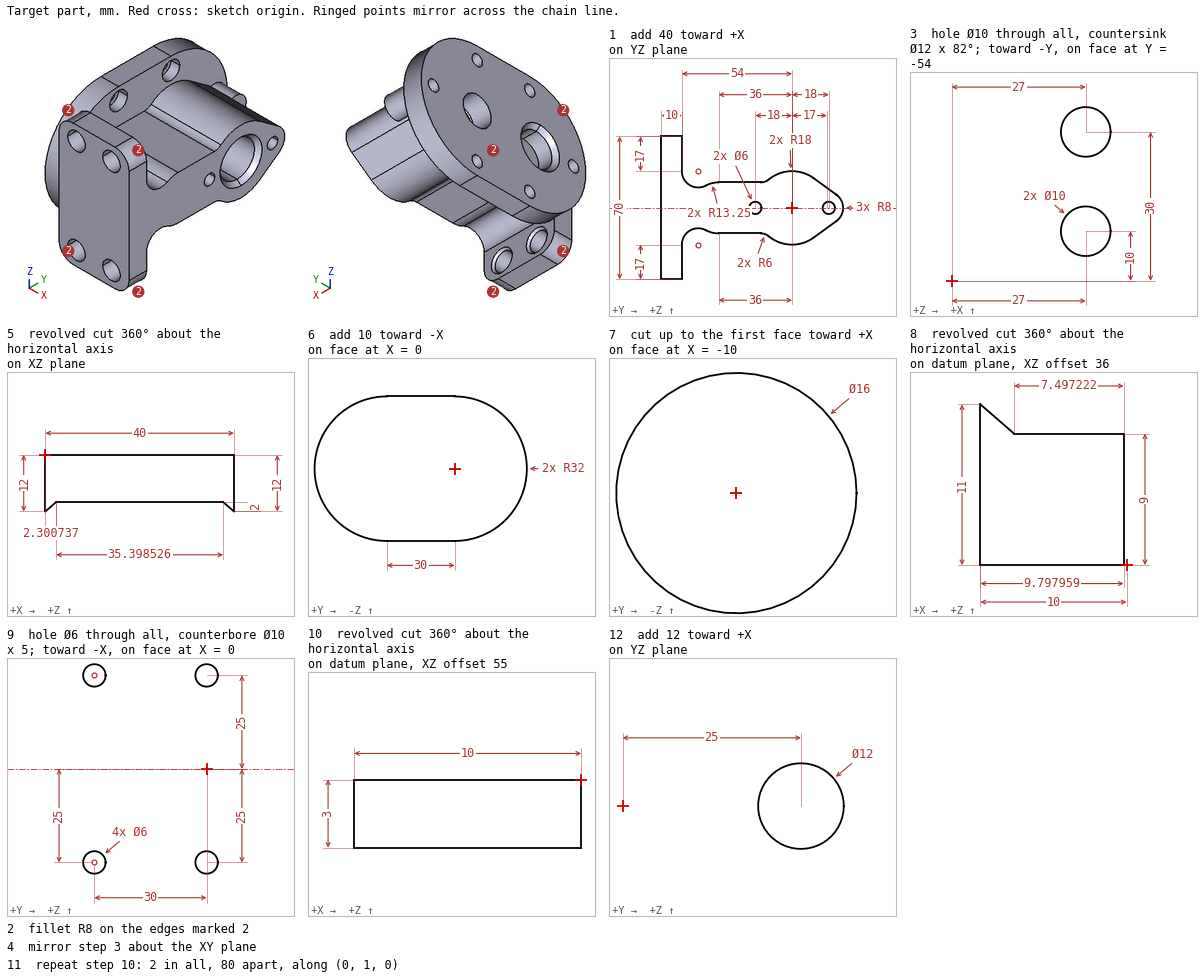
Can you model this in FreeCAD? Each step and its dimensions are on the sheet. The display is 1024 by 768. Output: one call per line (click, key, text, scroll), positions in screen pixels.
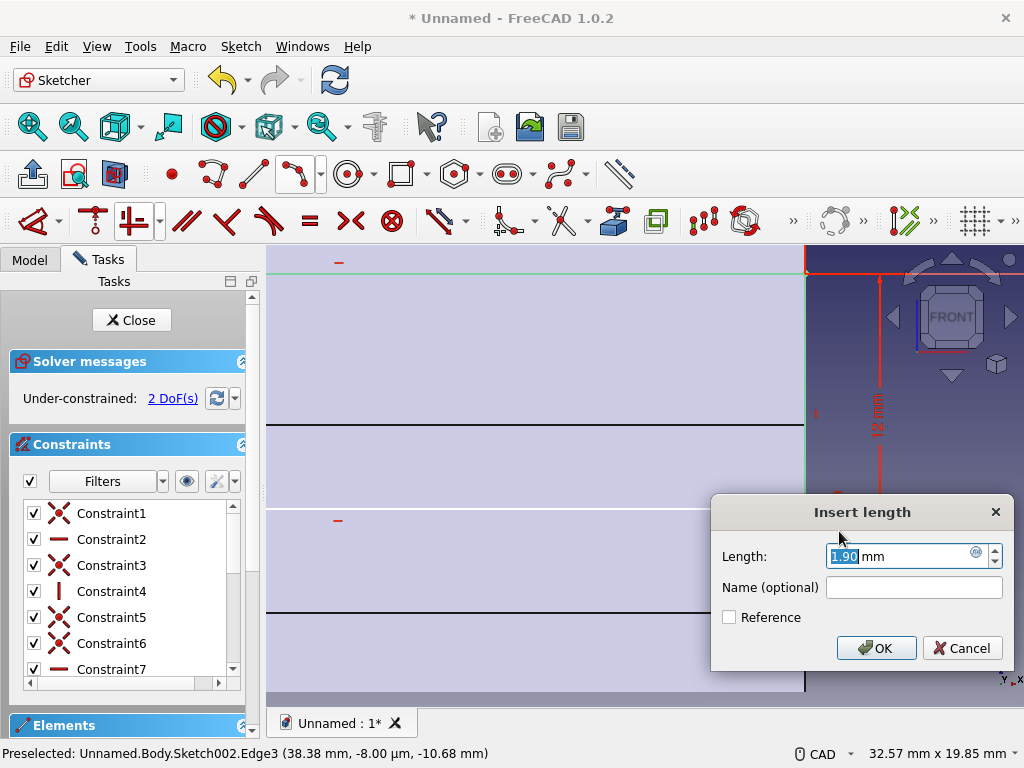
text(2)
key(Return)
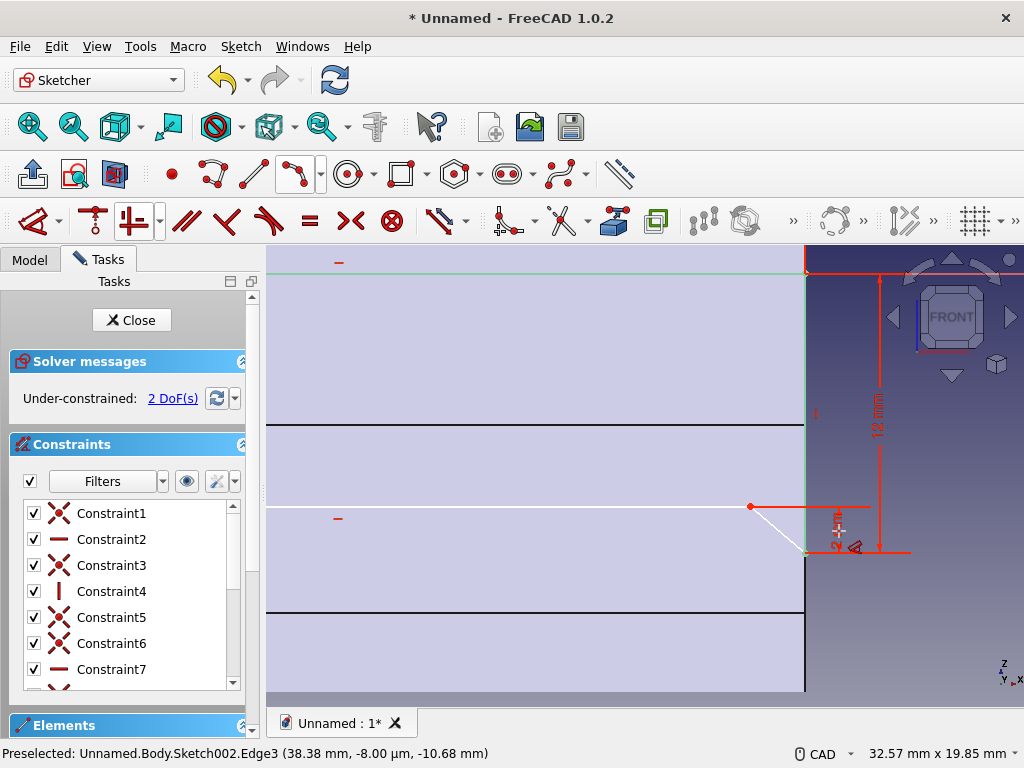
click(504, 507)
click(522, 541)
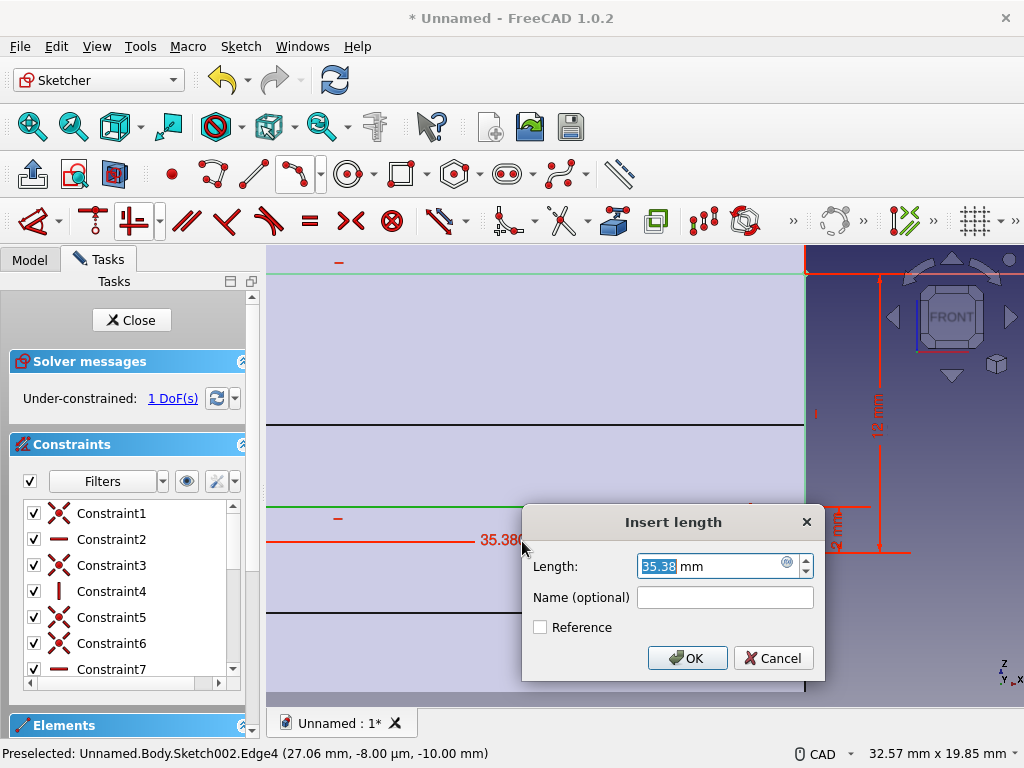
text(35.398526)
key(Return)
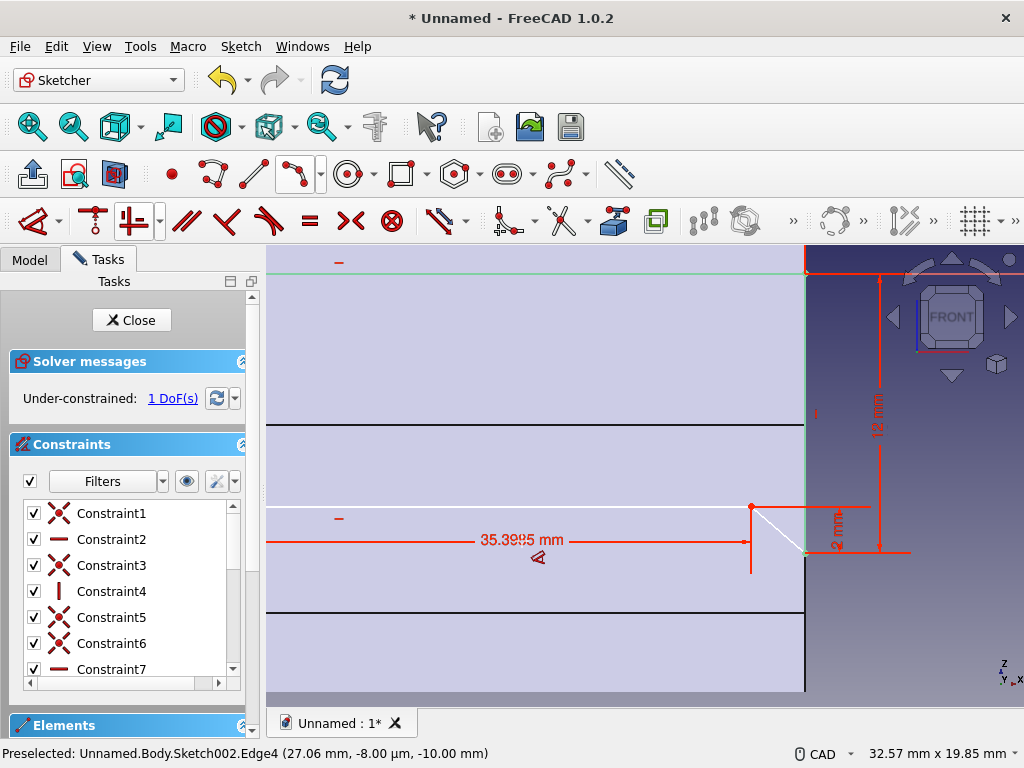
scroll(770, 527, down, 4)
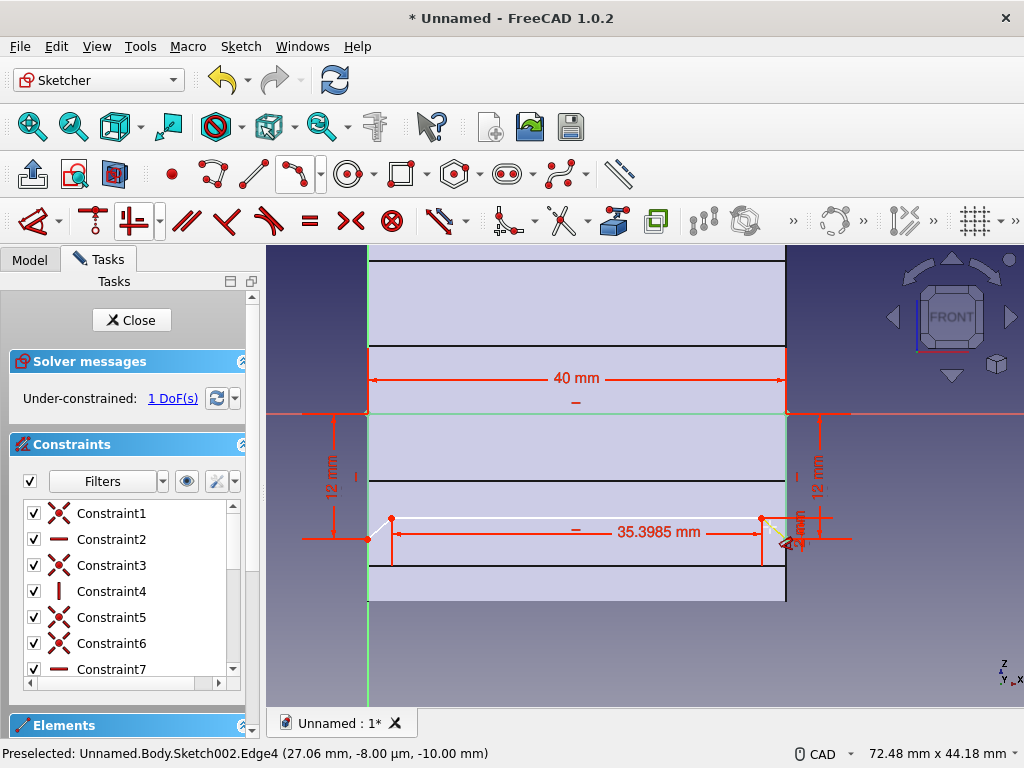
scroll(392, 518, up, 3)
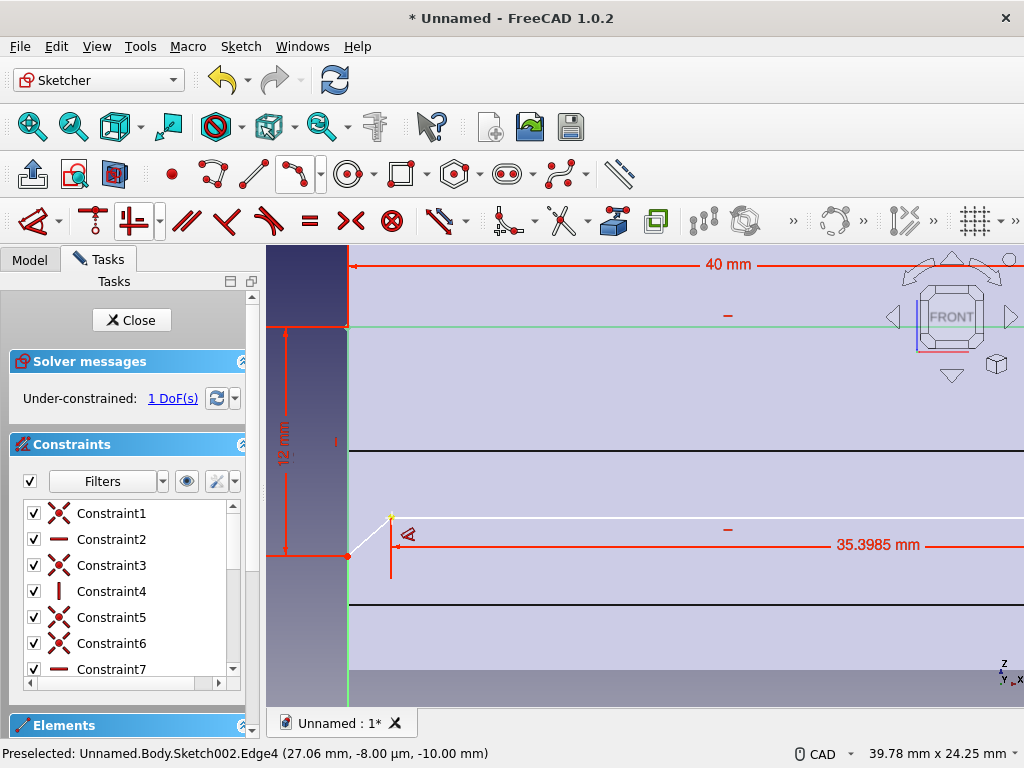
click(391, 518)
click(370, 293)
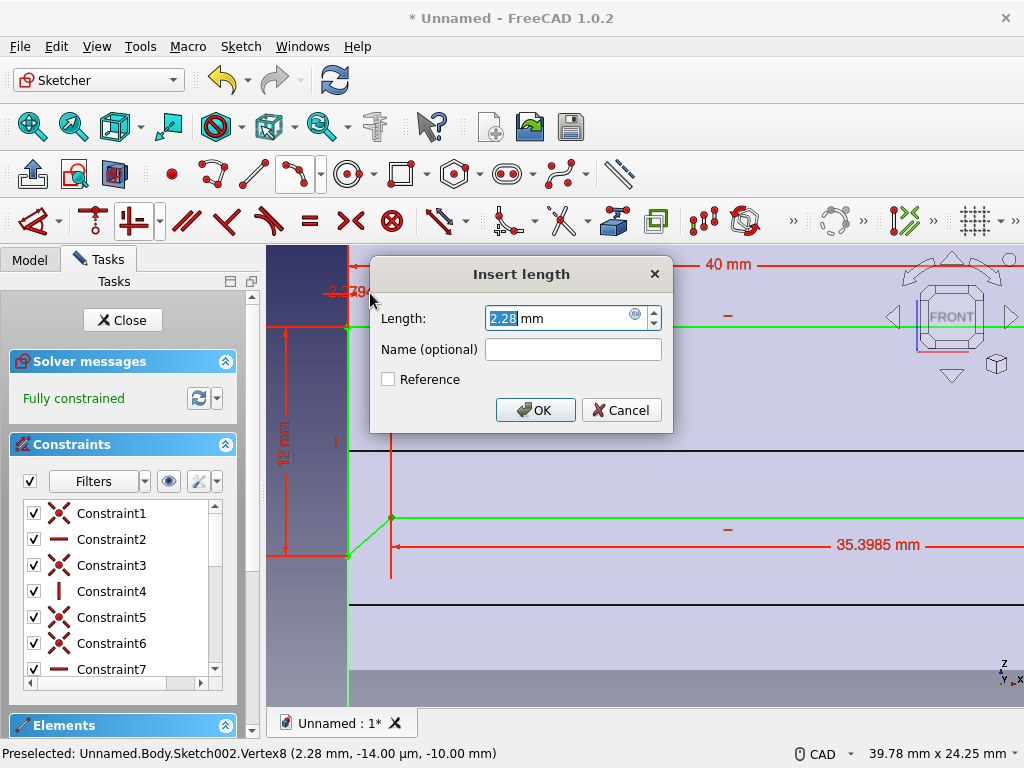
text(2.300737)
key(Return)
key(Escape)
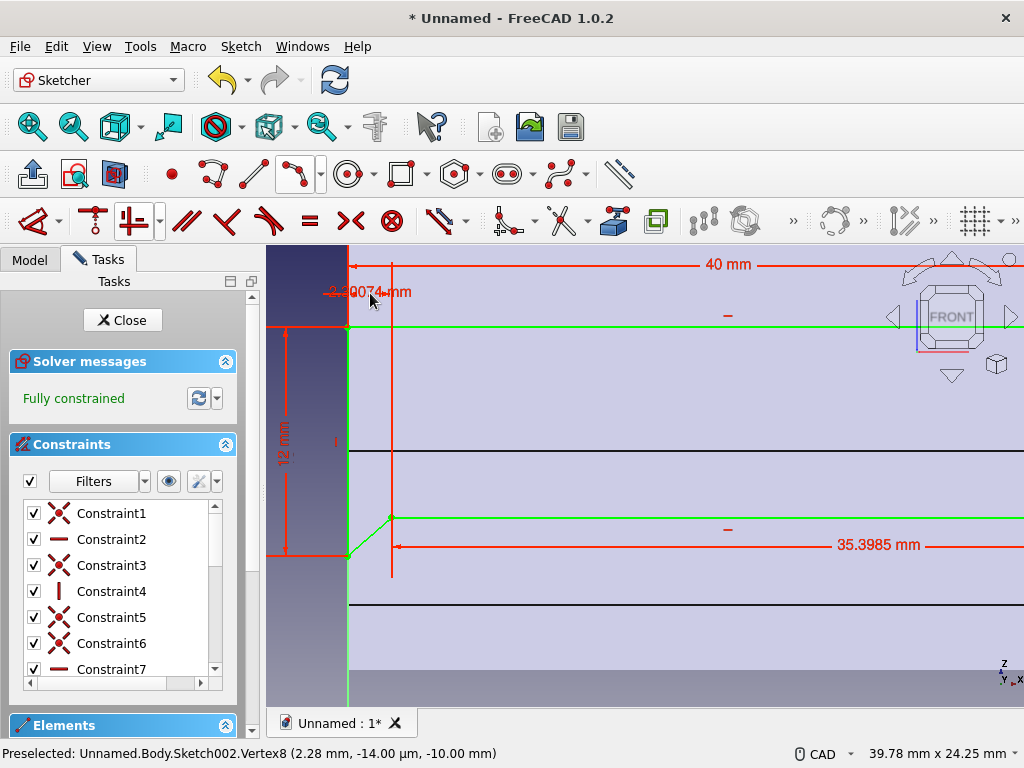
click(123, 320)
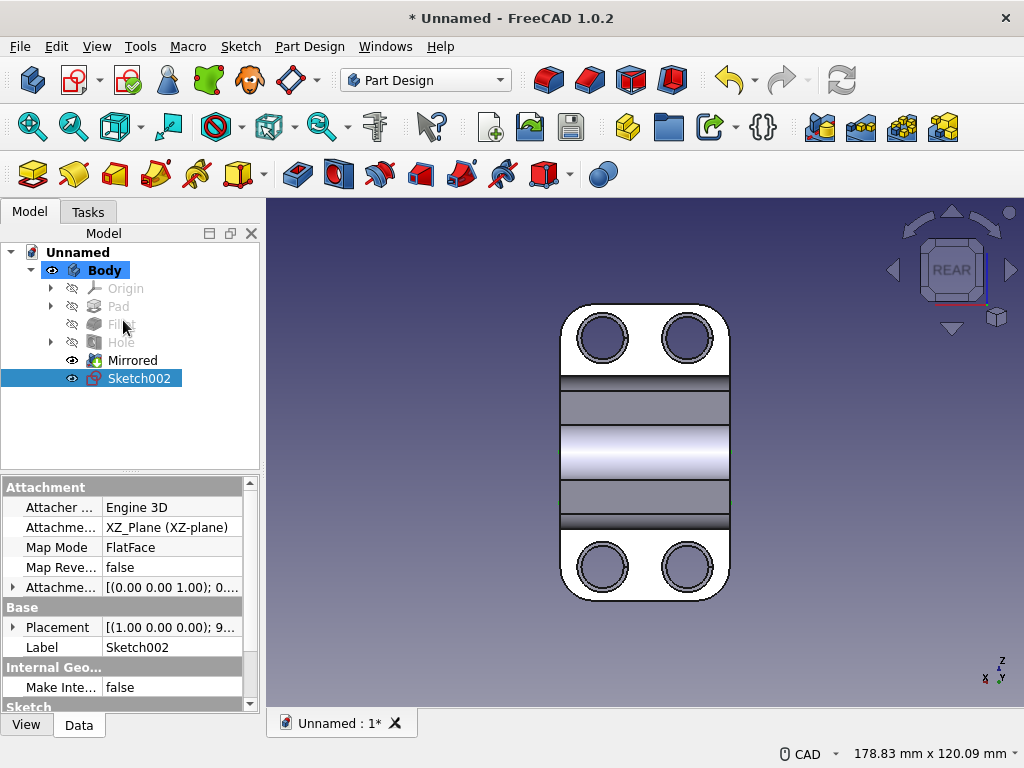
click(380, 174)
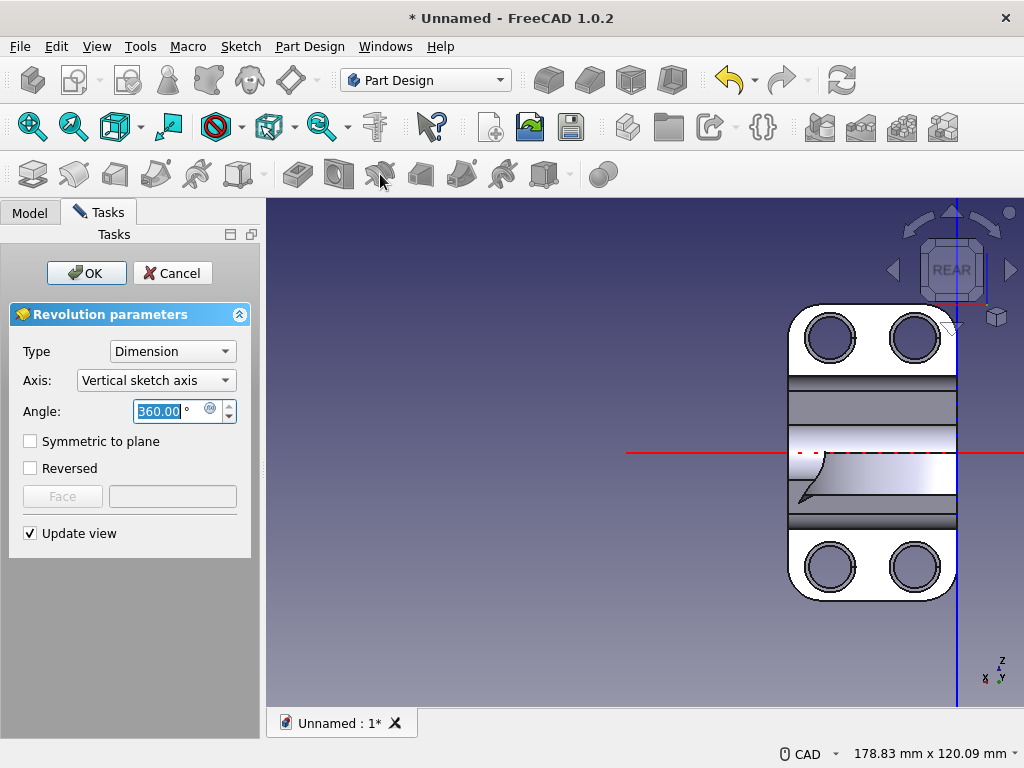
click(157, 380)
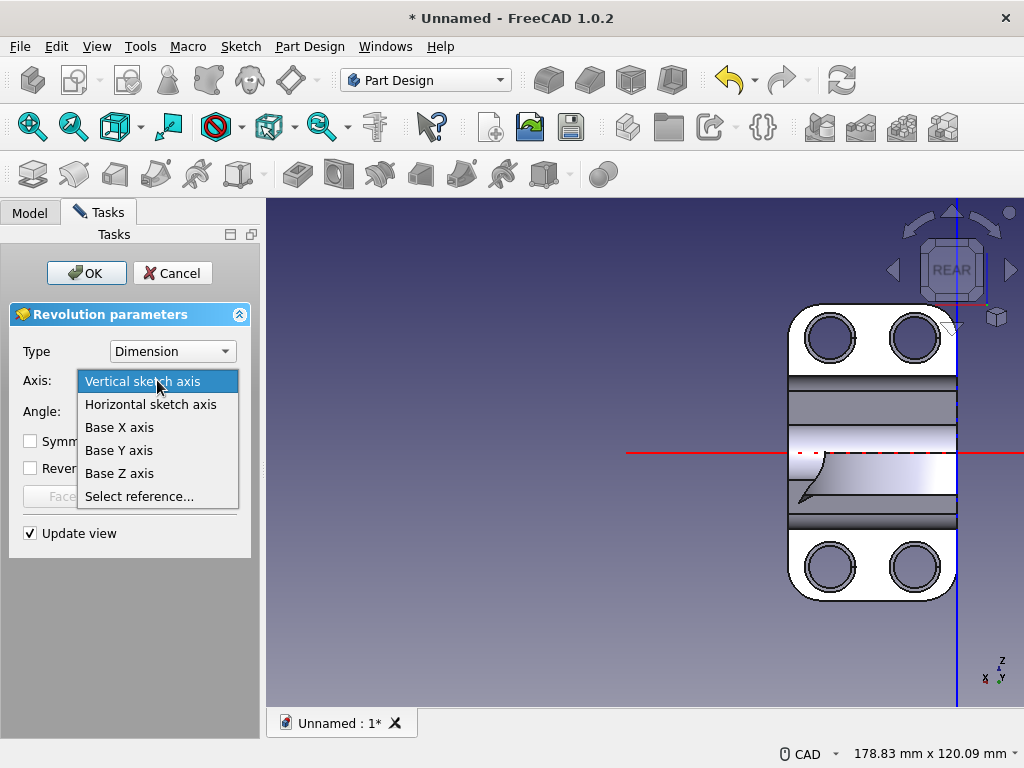
click(156, 404)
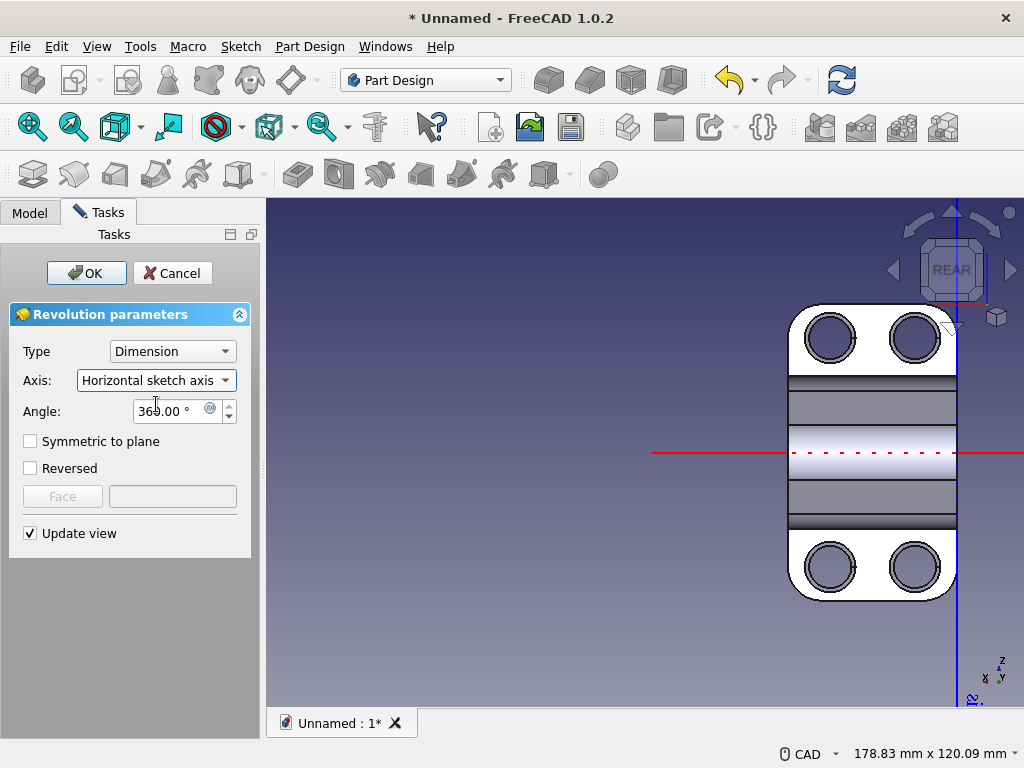
click(87, 273)